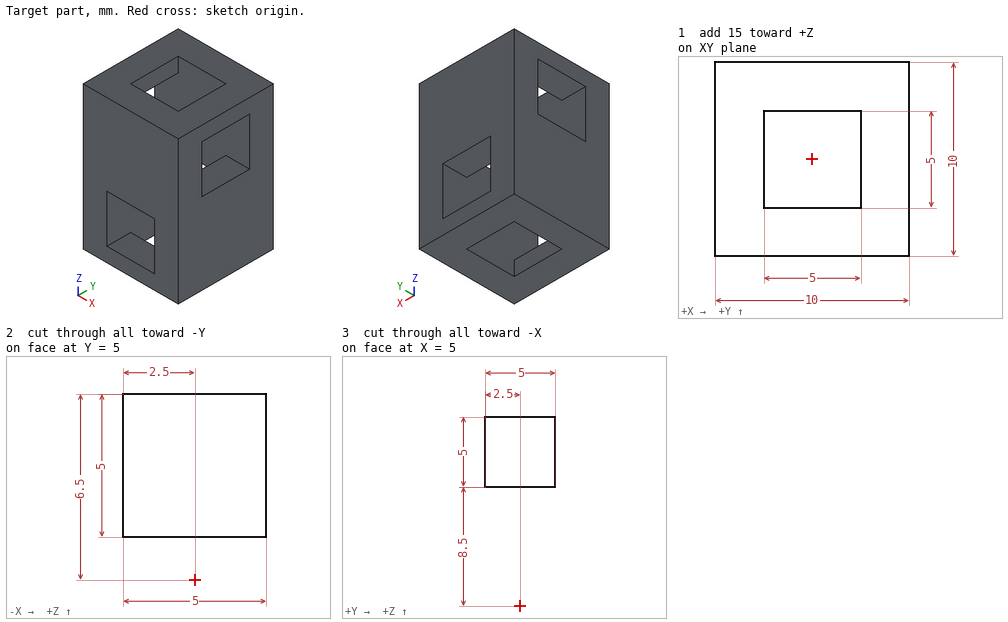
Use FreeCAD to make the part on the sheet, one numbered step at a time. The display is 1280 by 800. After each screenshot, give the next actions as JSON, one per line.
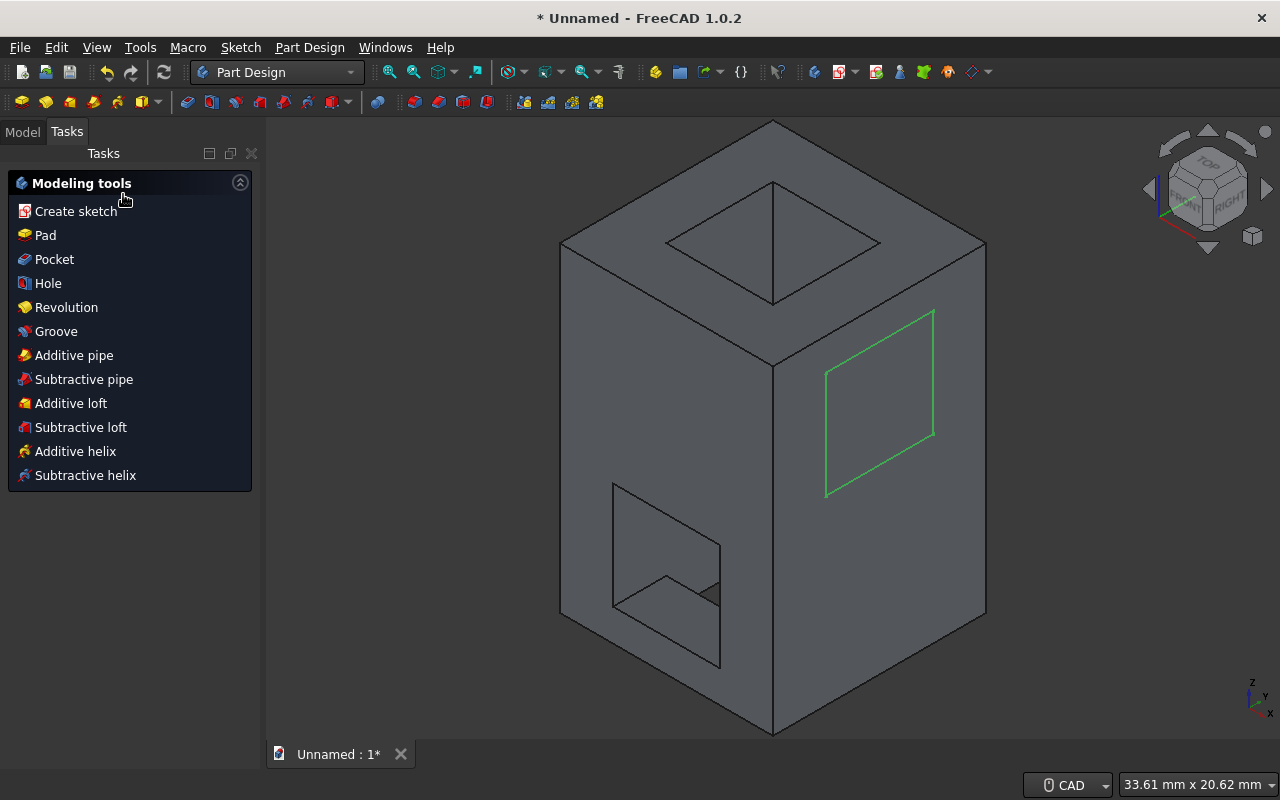
{"action": "left_click", "coordinate": [188, 102]}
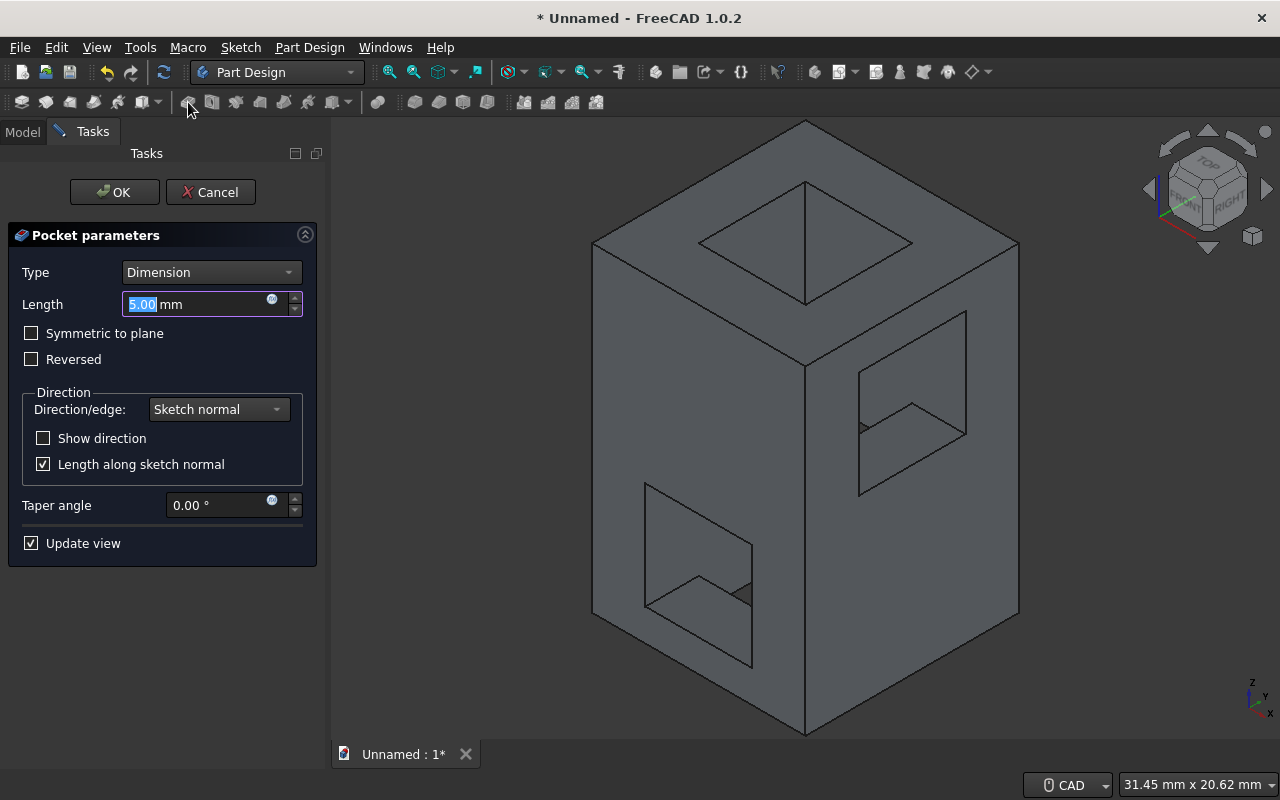
{"action": "left_click", "coordinate": [212, 272]}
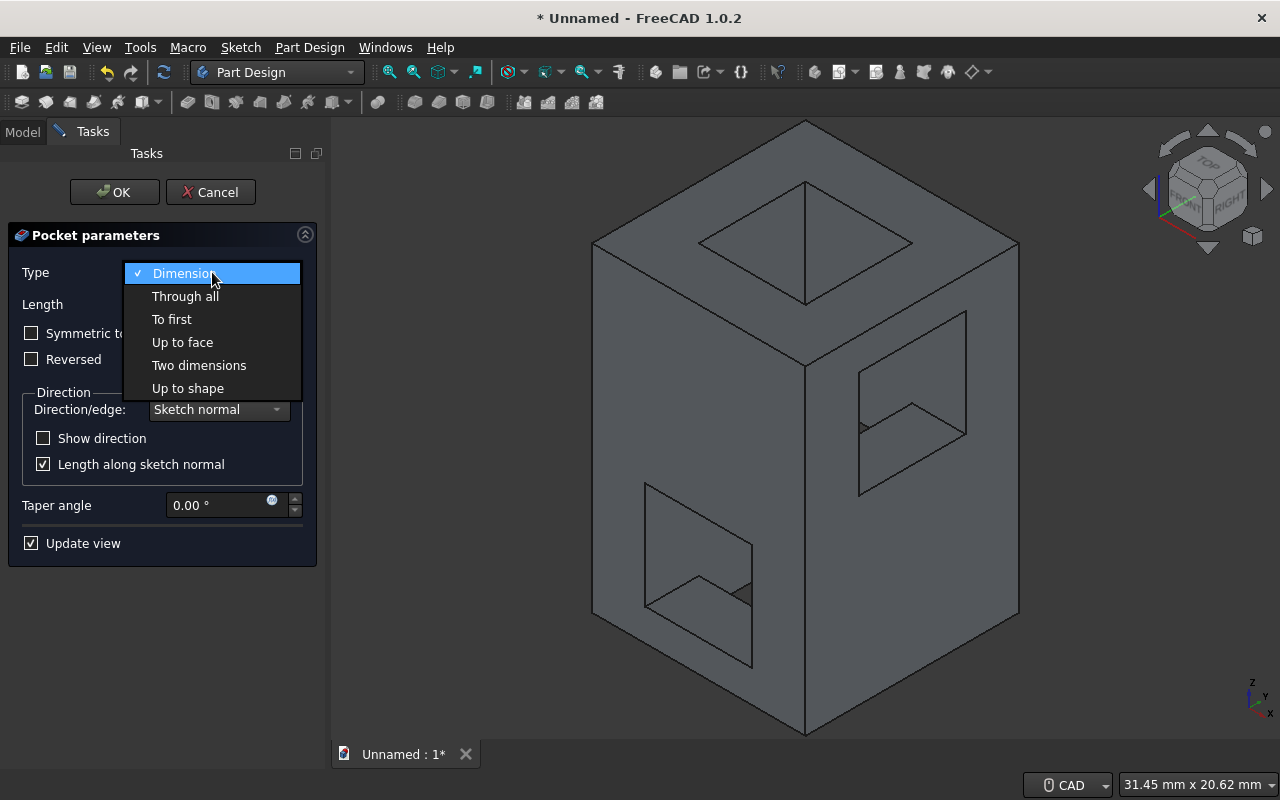
{"action": "left_click", "coordinate": [212, 296]}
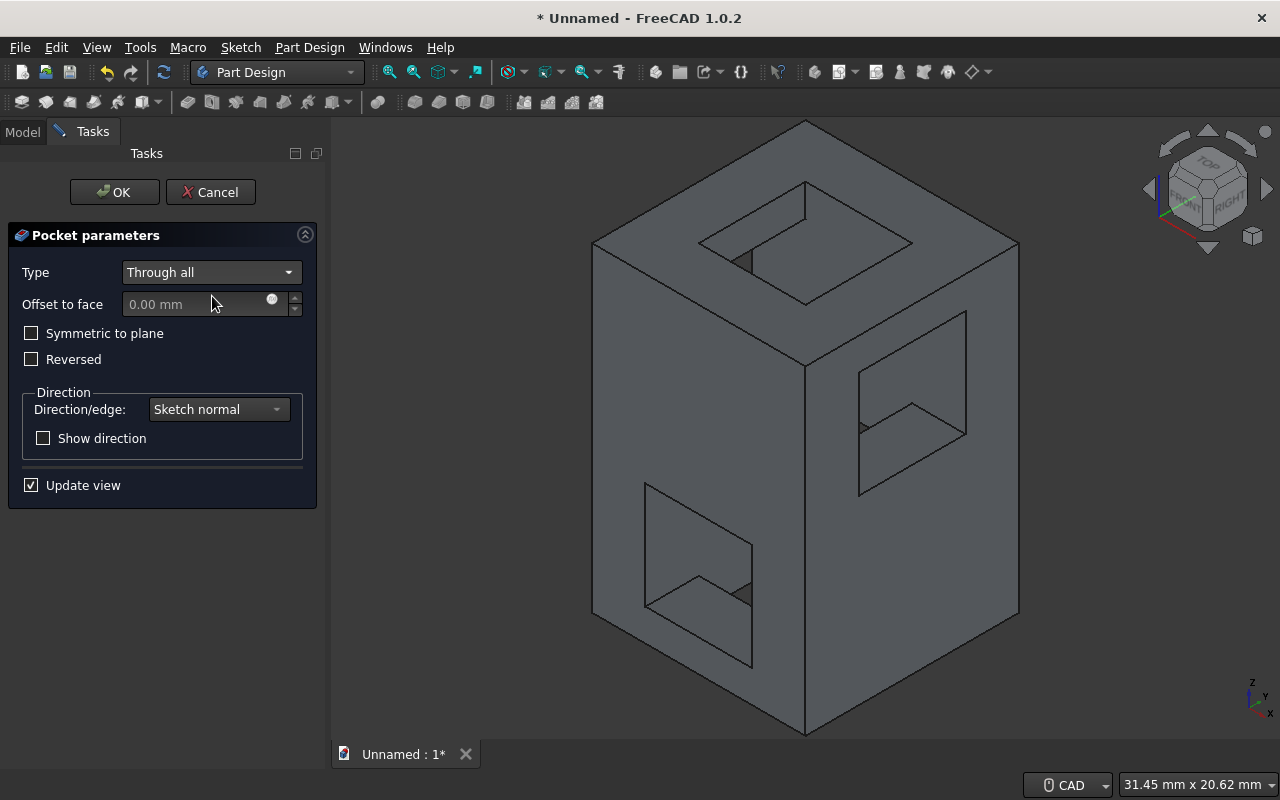
{"action": "left_click", "coordinate": [115, 192]}